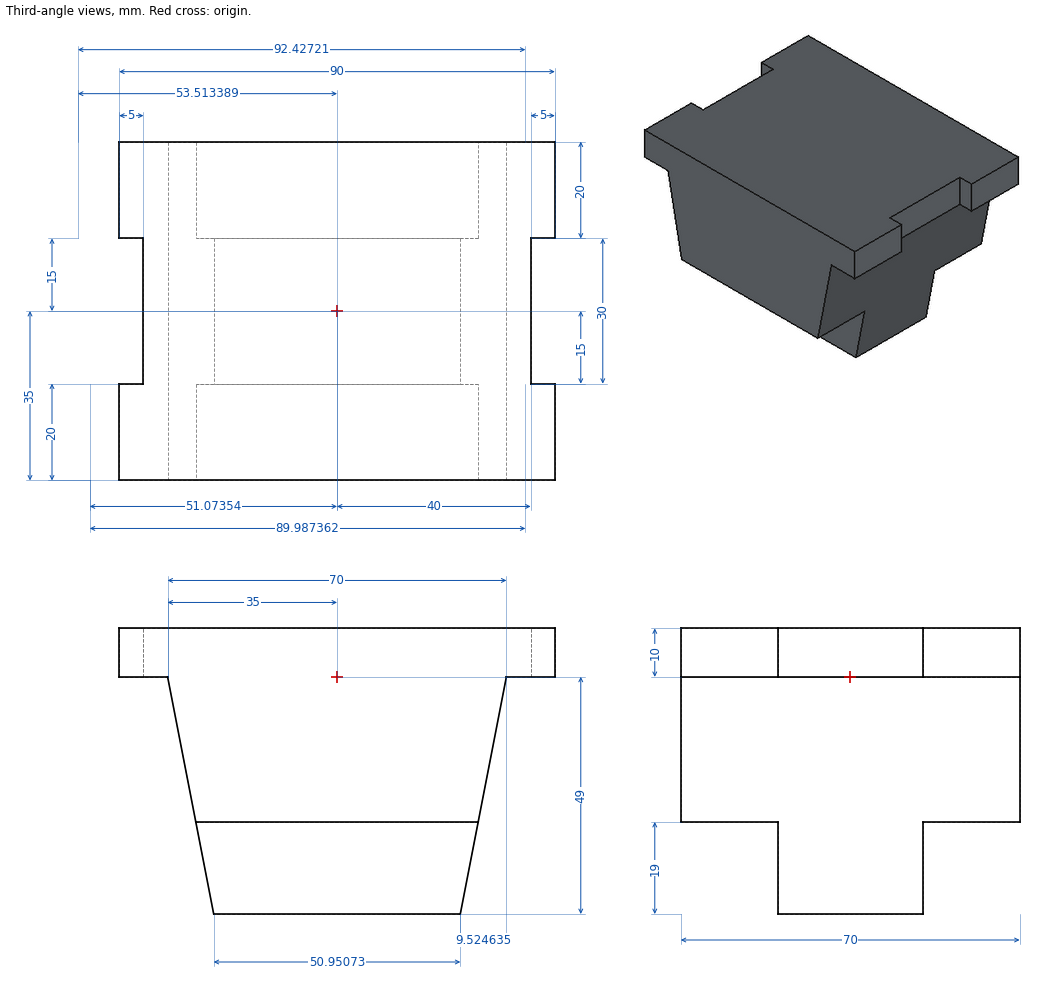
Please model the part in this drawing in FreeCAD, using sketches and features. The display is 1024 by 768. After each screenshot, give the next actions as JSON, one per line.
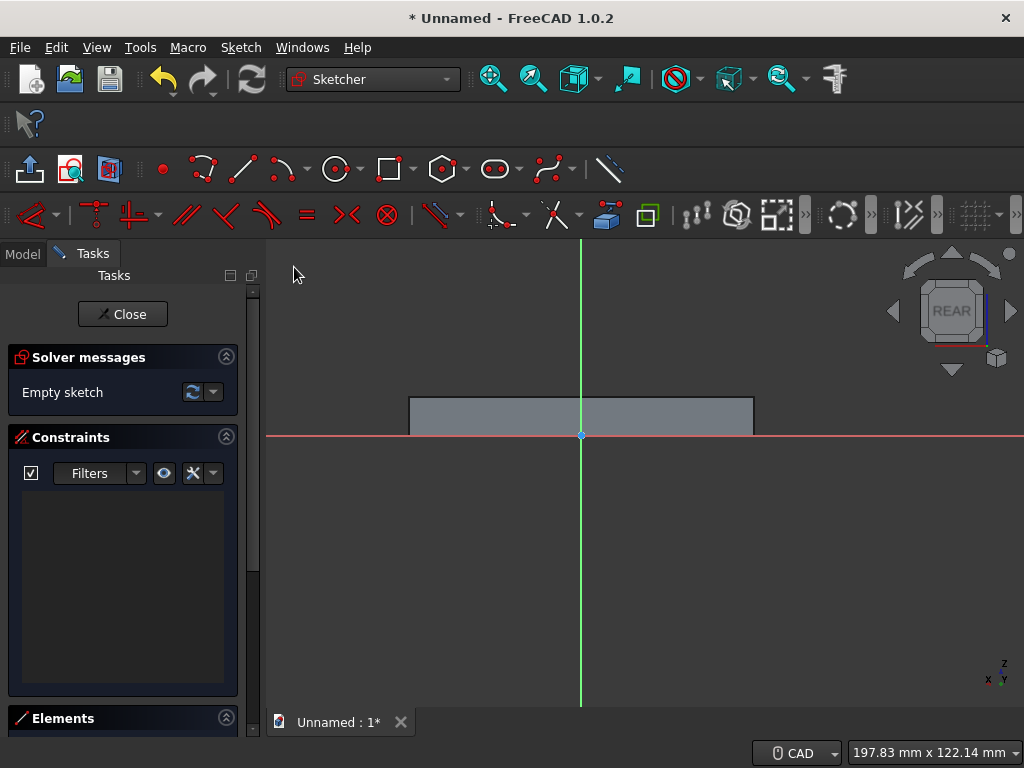
{"action": "scroll", "coordinate": [591, 645], "scroll_direction": "up", "scroll_amount": 2}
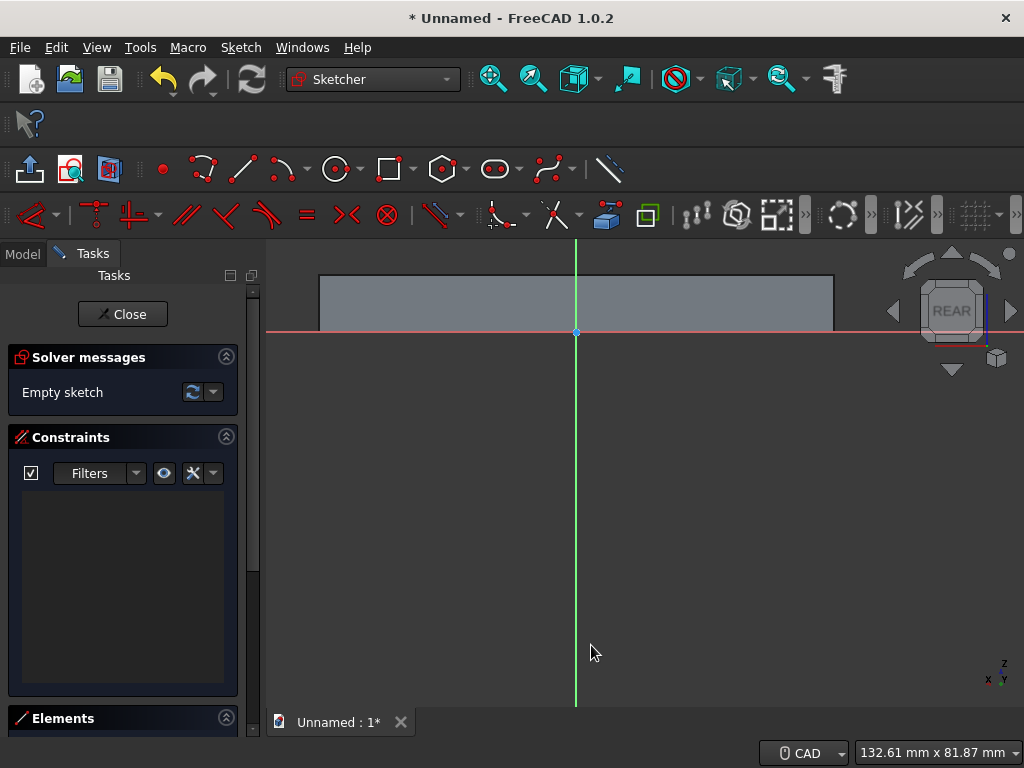
{"action": "left_click", "coordinate": [204, 170]}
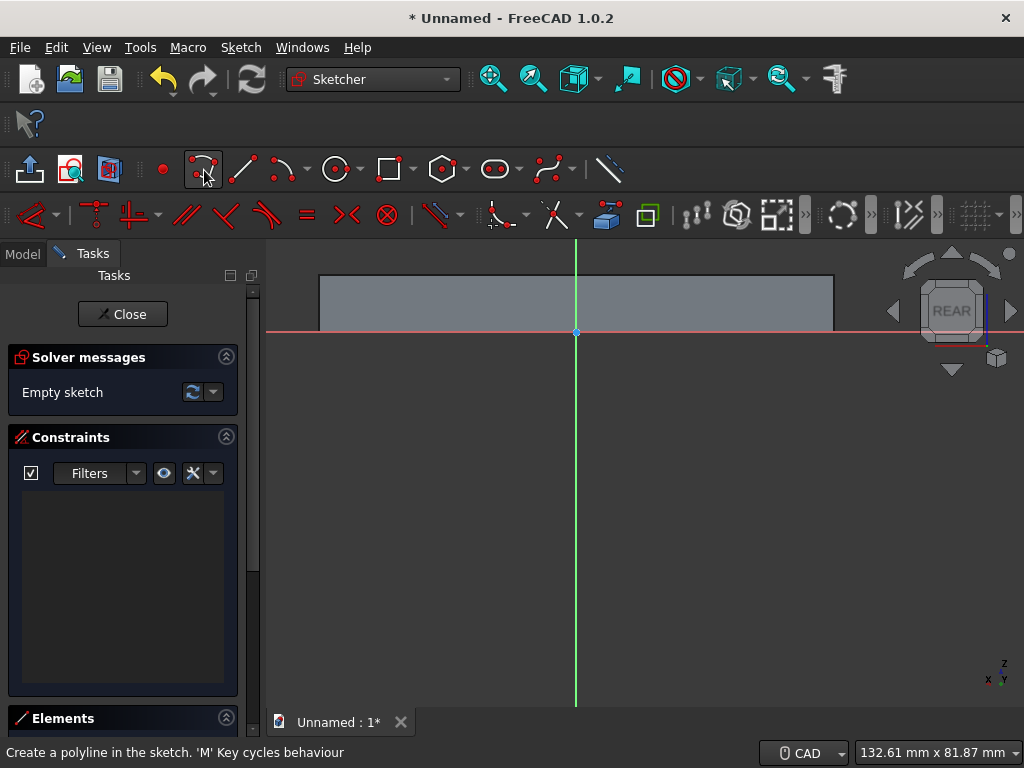
{"action": "left_click", "coordinate": [777, 332]}
{"action": "left_click", "coordinate": [376, 341]}
{"action": "left_click", "coordinate": [431, 612]}
{"action": "left_click", "coordinate": [722, 612]}
{"action": "left_click", "coordinate": [777, 332]}
{"action": "key", "text": "Escape"}
{"action": "key", "text": "Escape"}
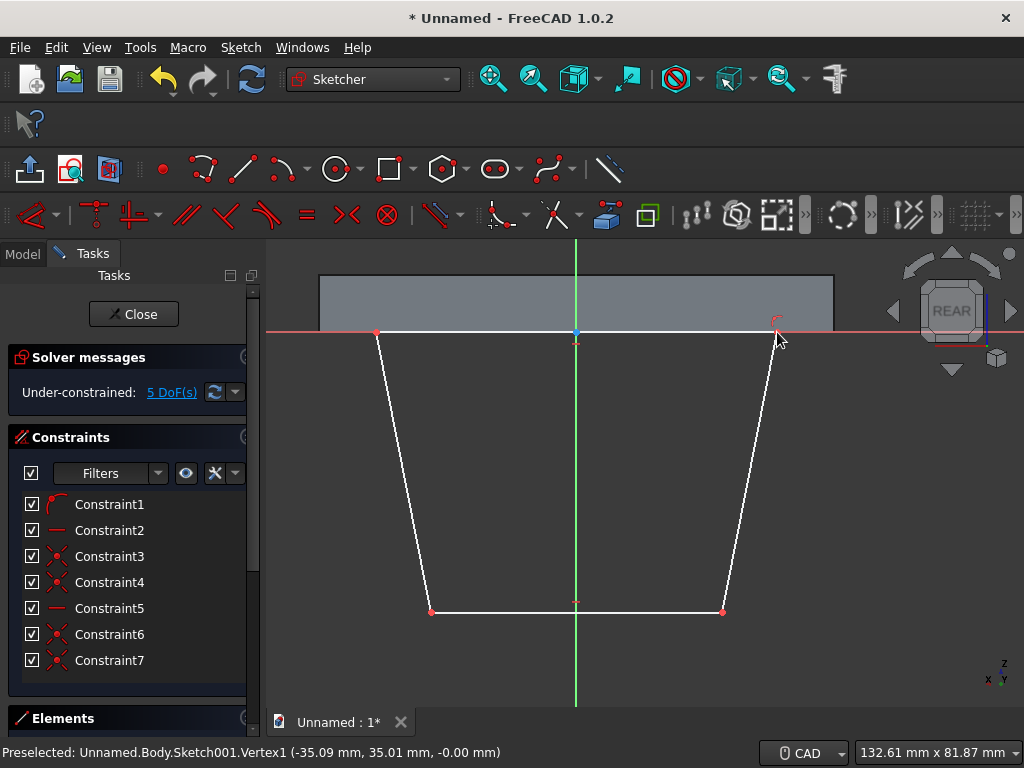
{"action": "left_click", "coordinate": [32, 216]}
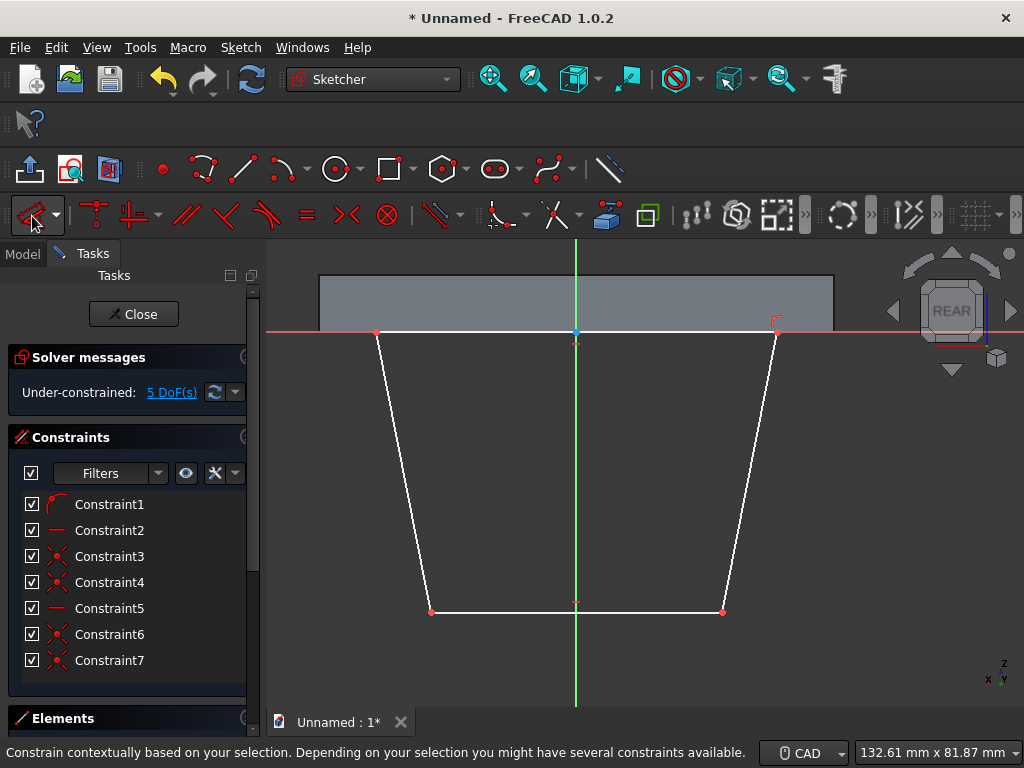
{"action": "left_click", "coordinate": [657, 332]}
{"action": "left_click", "coordinate": [484, 298]}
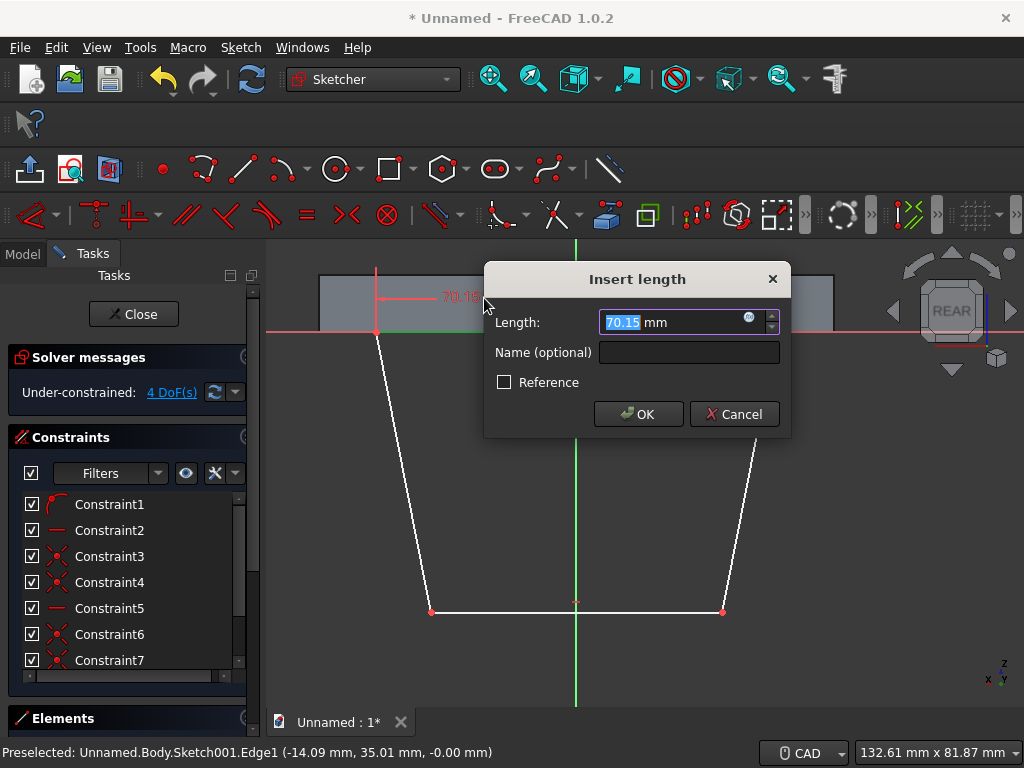
{"action": "type", "text": "70"}
{"action": "key", "text": "Return"}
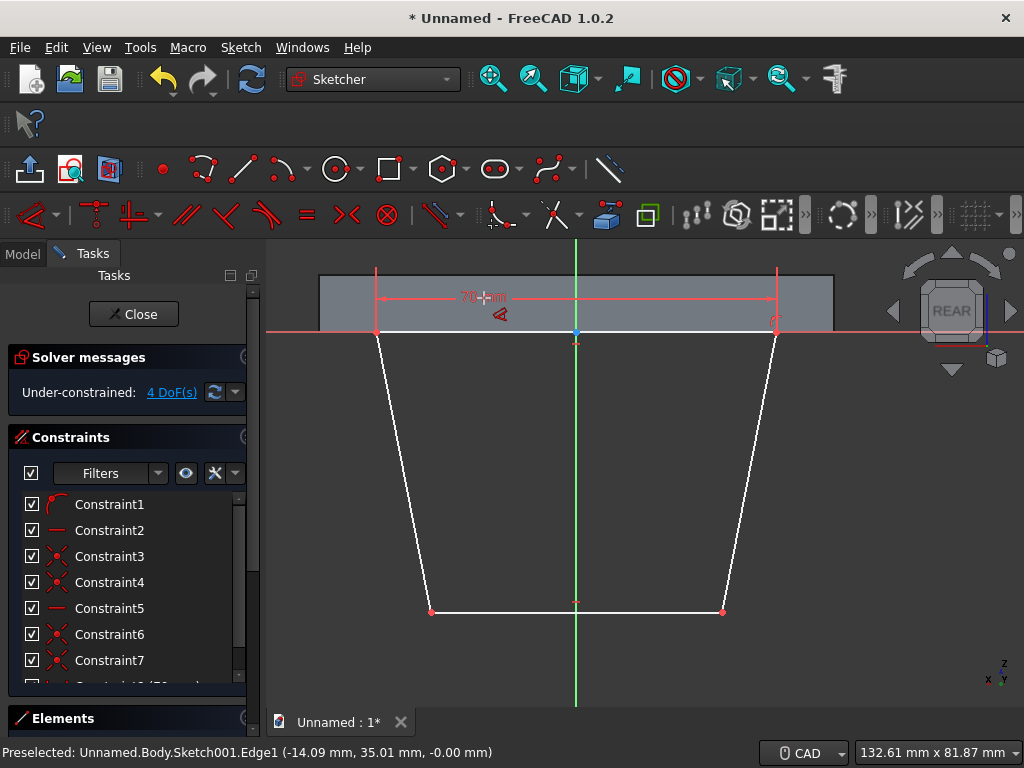
{"action": "left_click", "coordinate": [777, 332]}
{"action": "left_click", "coordinate": [676, 298]}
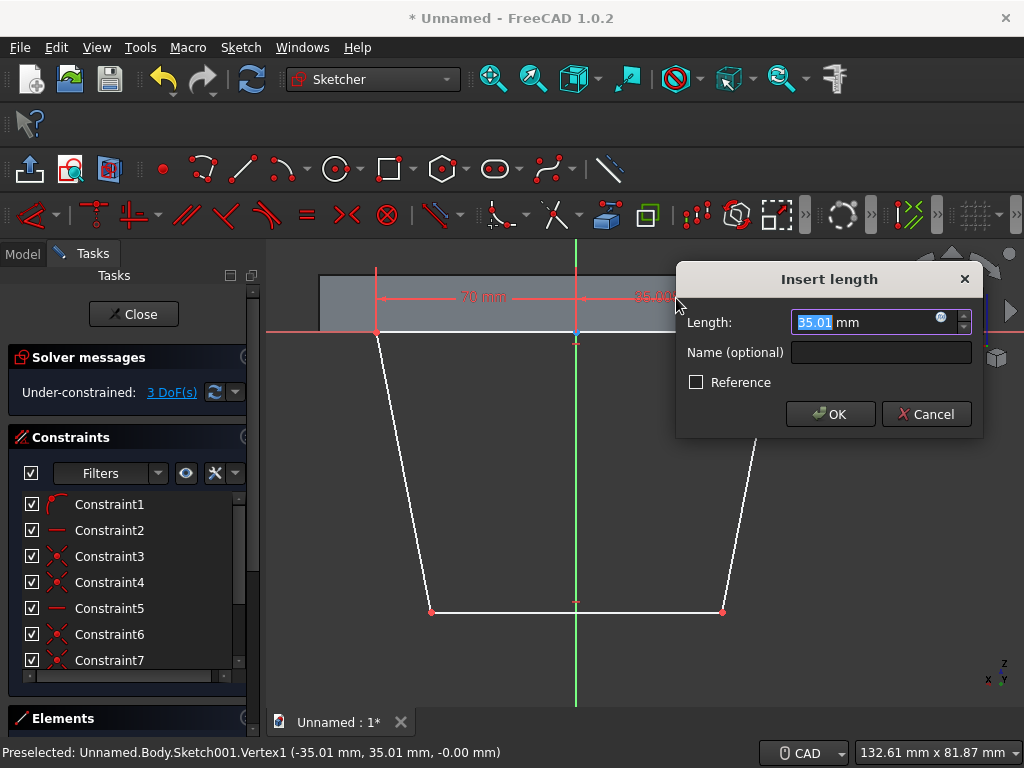
{"action": "type", "text": "35"}
{"action": "key", "text": "Return"}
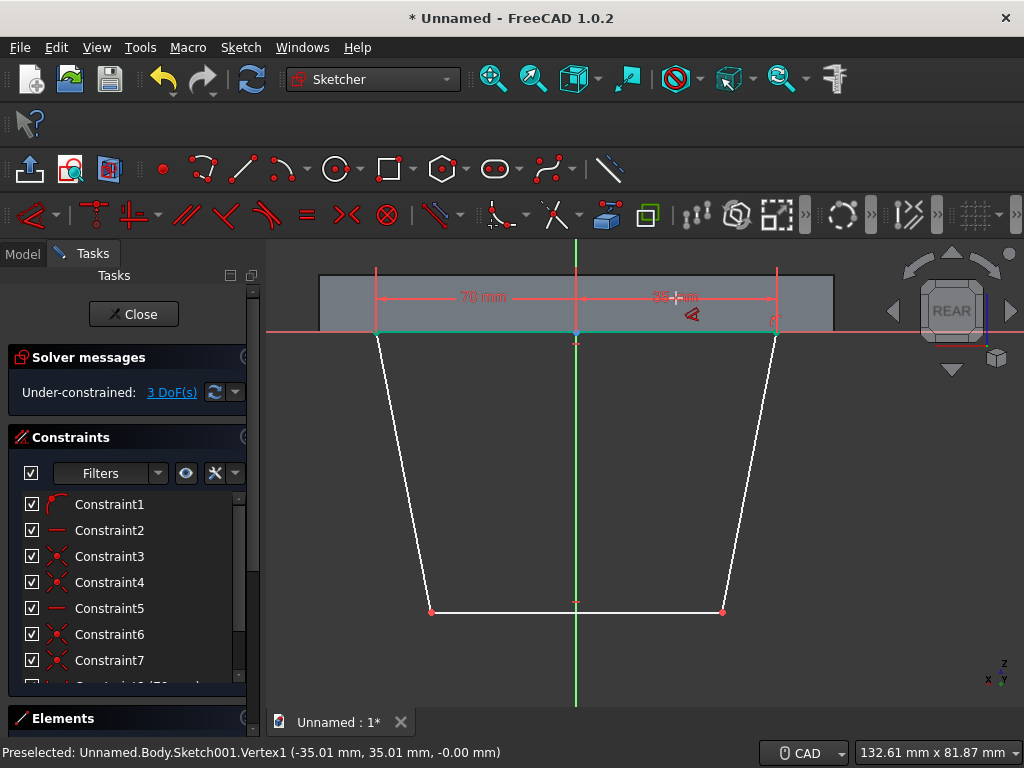
{"action": "left_click", "coordinate": [431, 613]}
{"action": "left_click", "coordinate": [397, 537]}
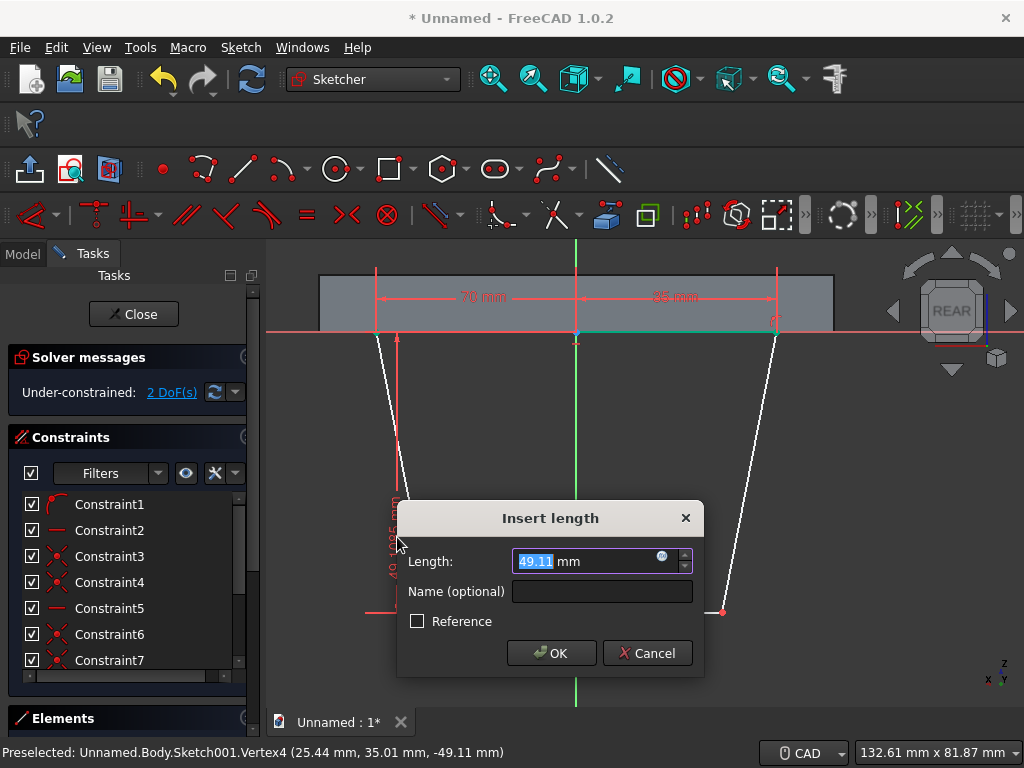
{"action": "type", "text": "49"}
{"action": "key", "text": "Return"}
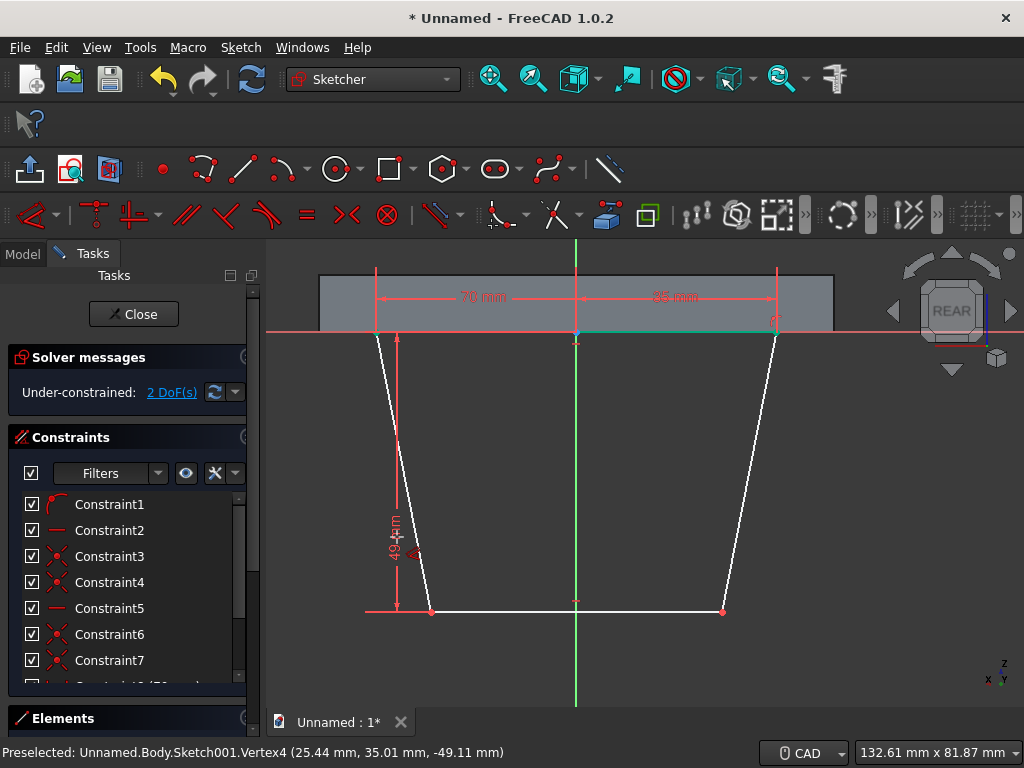
{"action": "left_click", "coordinate": [518, 612]}
{"action": "left_click", "coordinate": [510, 646]}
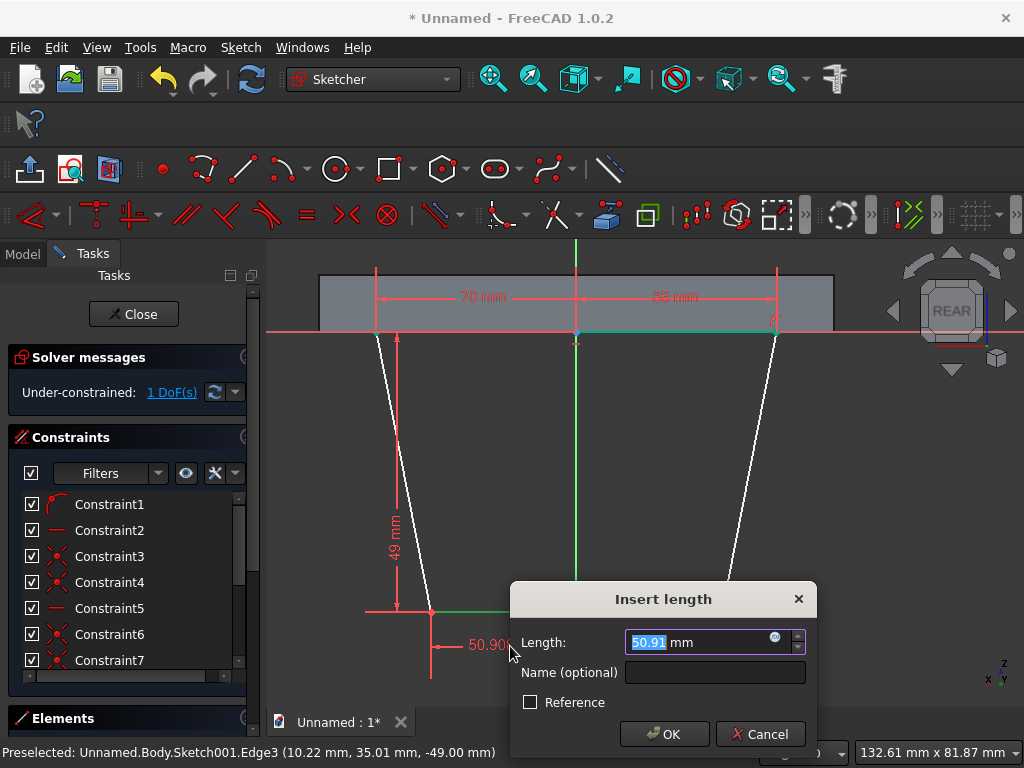
{"action": "type", "text": "50.95073"}
{"action": "key", "text": "Return"}